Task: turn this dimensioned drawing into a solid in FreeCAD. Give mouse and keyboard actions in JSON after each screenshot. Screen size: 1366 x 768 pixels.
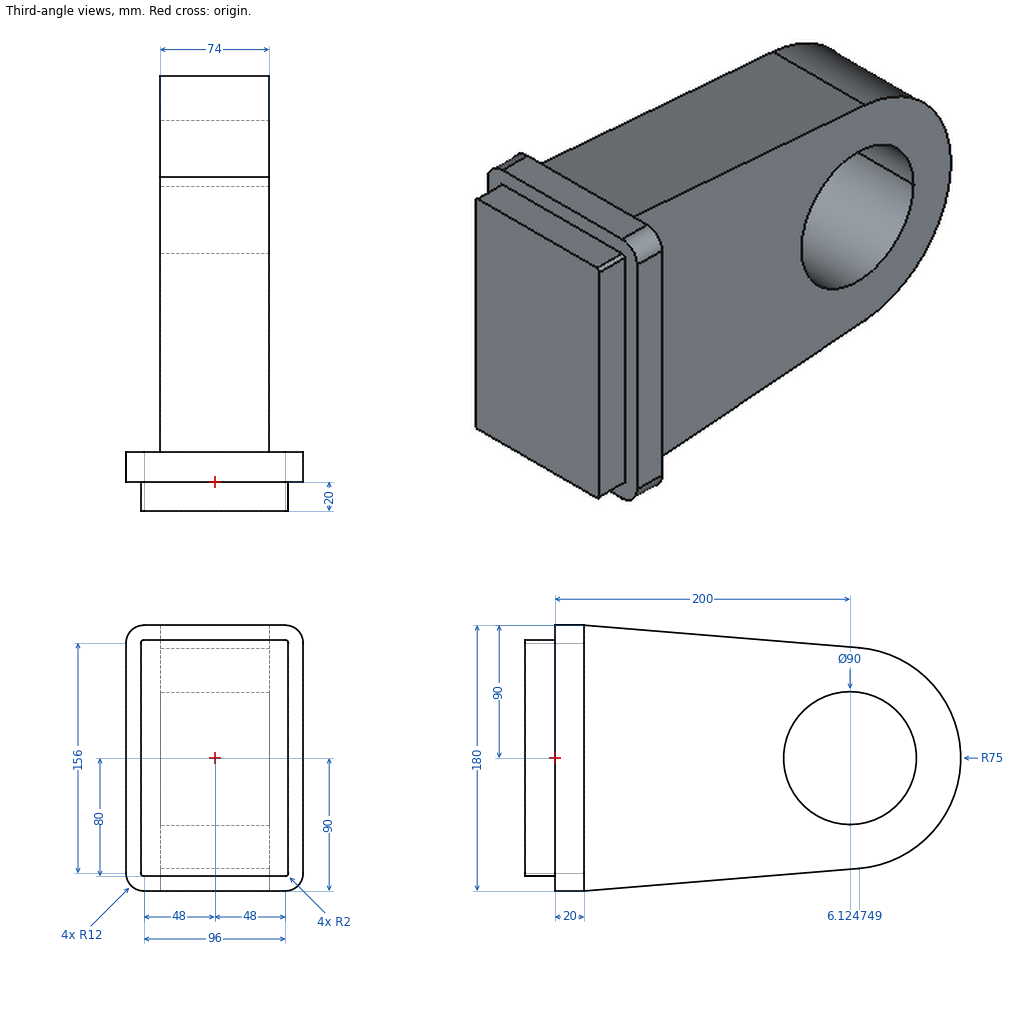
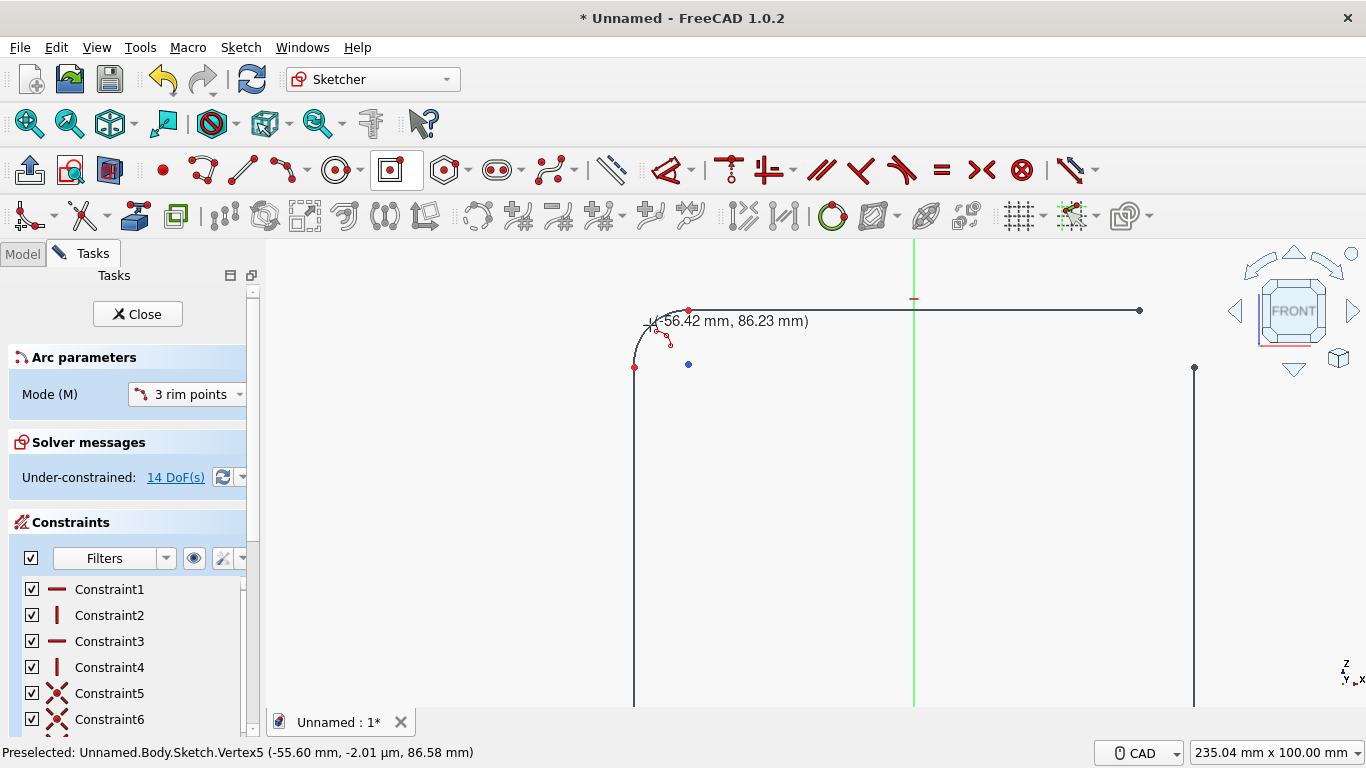
{"action": "left_click", "coordinate": [1140, 310]}
{"action": "left_click", "coordinate": [1194, 367]}
{"action": "left_click", "coordinate": [1178, 325]}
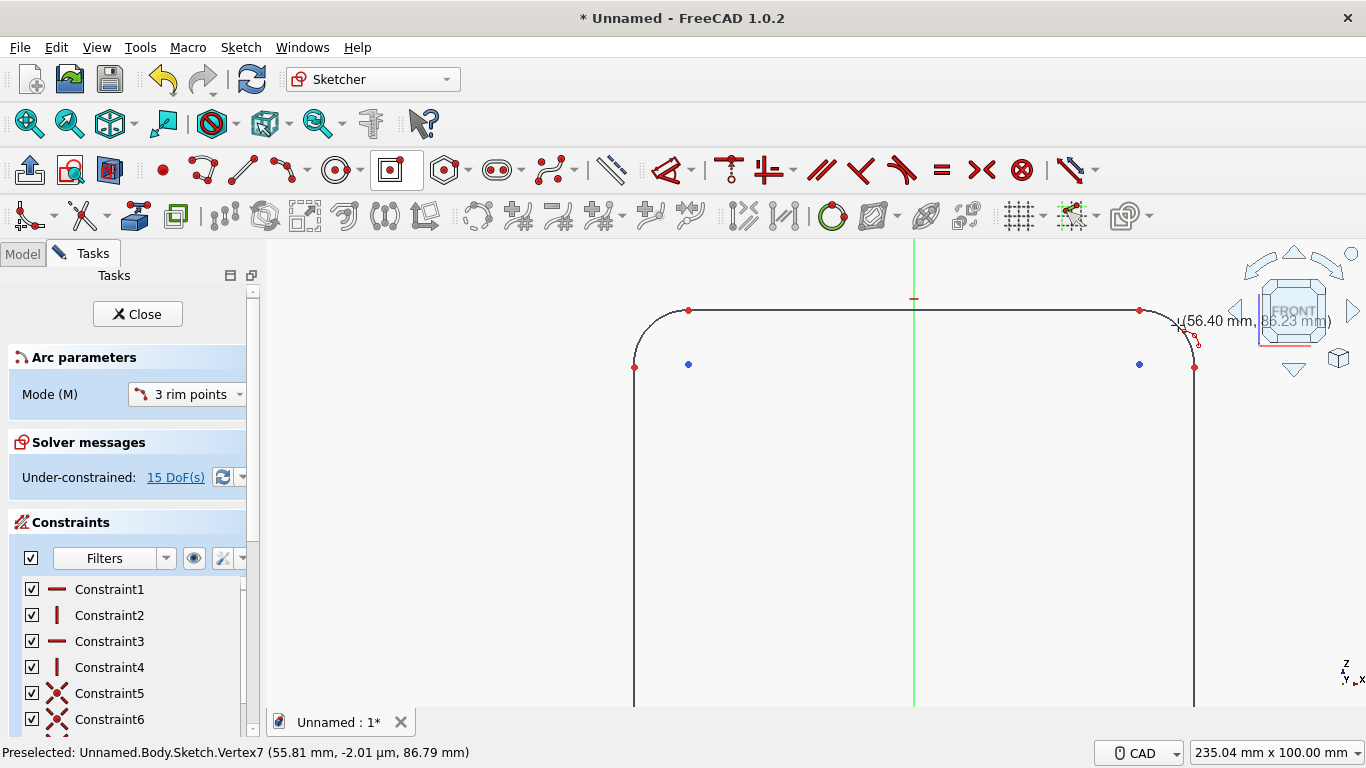
{"action": "scroll", "coordinate": [651, 324], "scroll_direction": "down", "scroll_amount": 5}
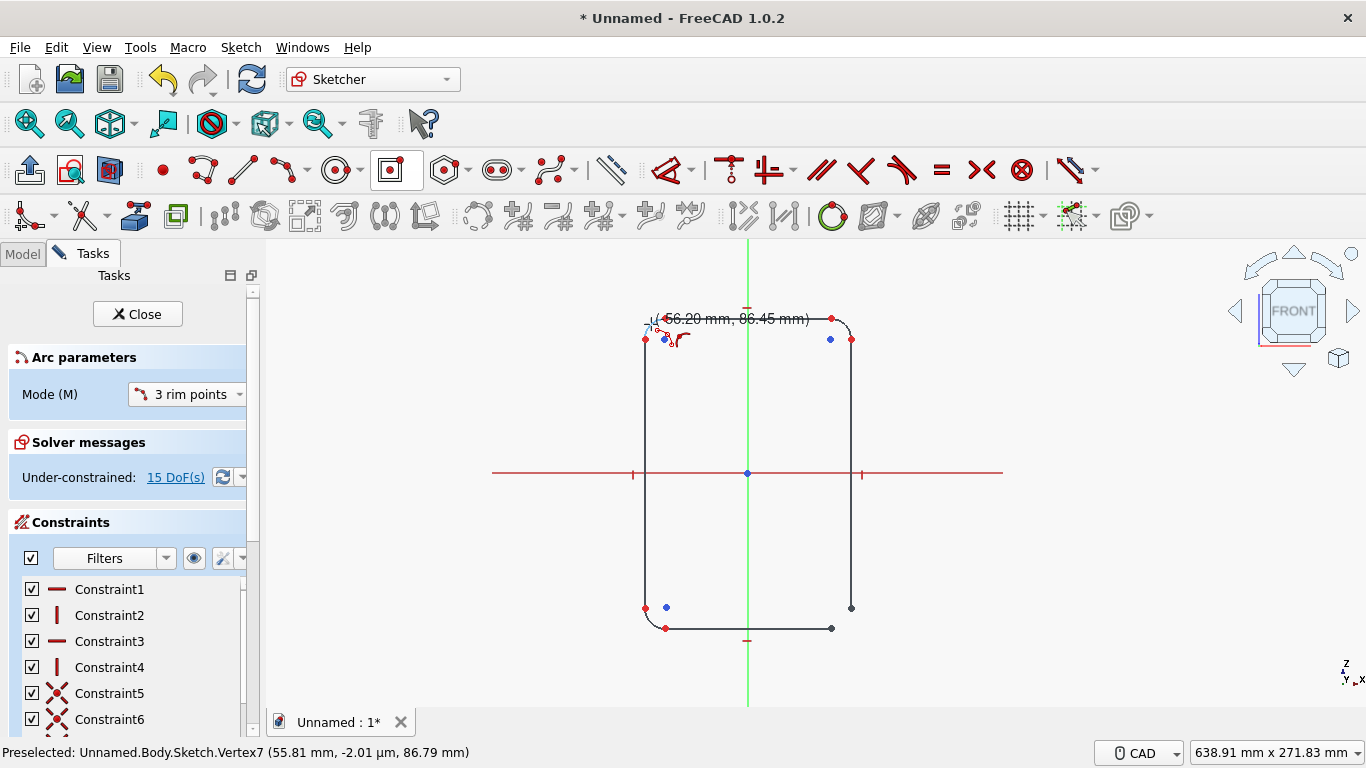
{"action": "left_click", "coordinate": [851, 609]}
{"action": "left_click", "coordinate": [831, 629]}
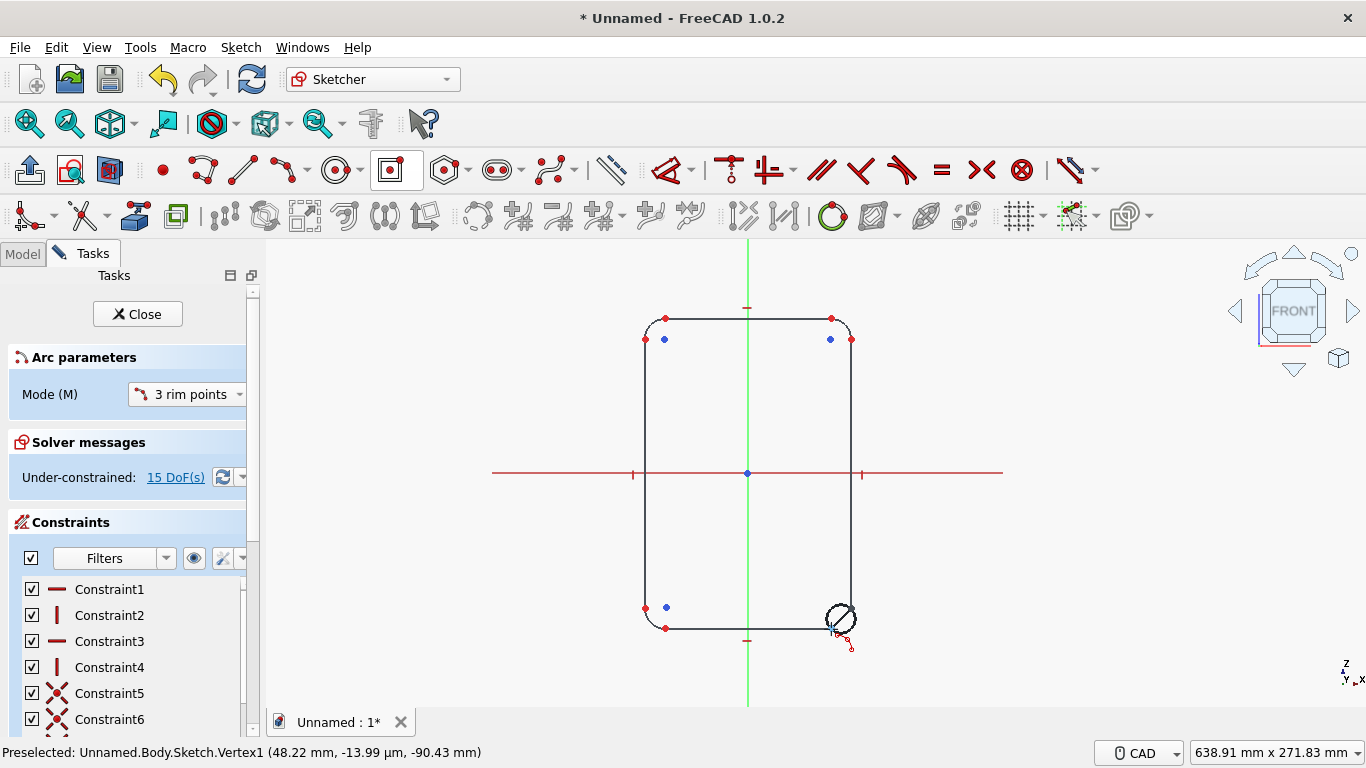
{"action": "scroll", "coordinate": [845, 622], "scroll_direction": "up", "scroll_amount": 5}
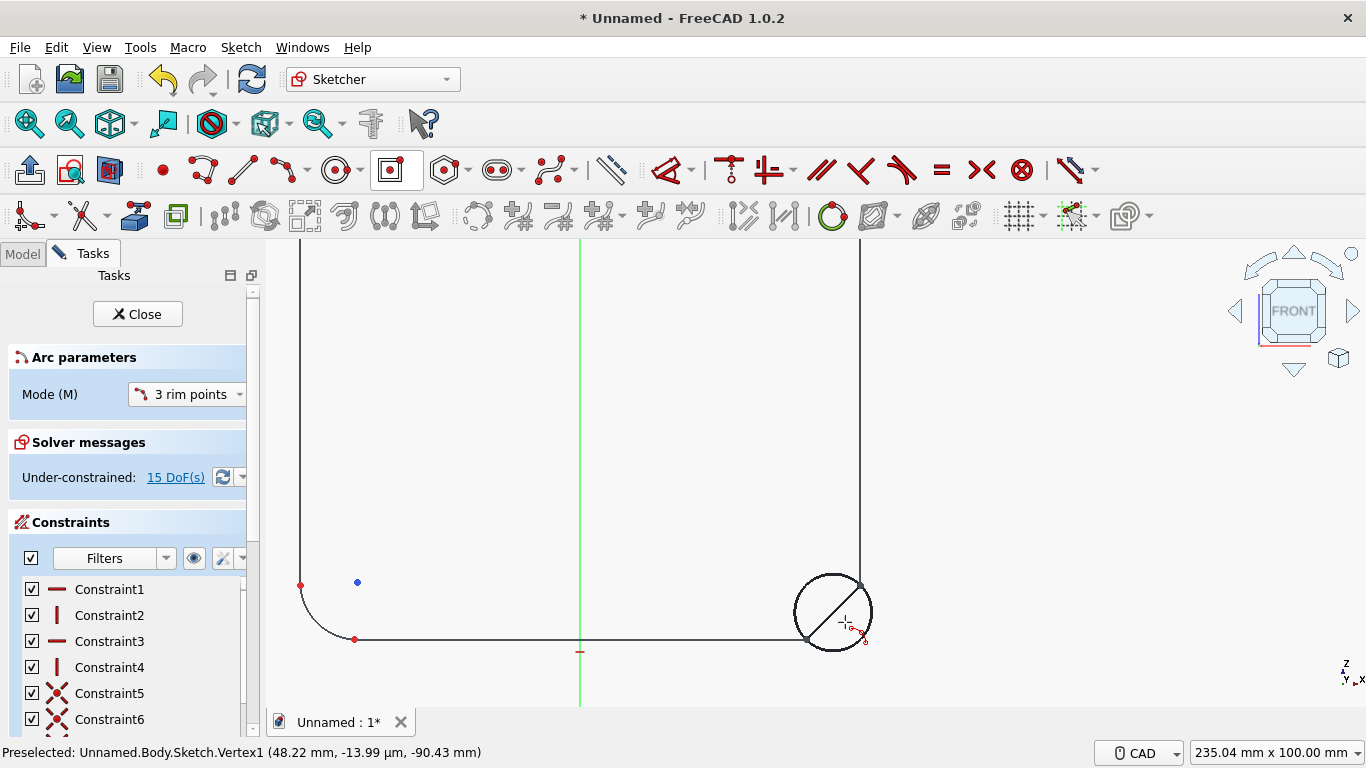
{"action": "left_click", "coordinate": [845, 621]}
{"action": "key", "text": "Escape"}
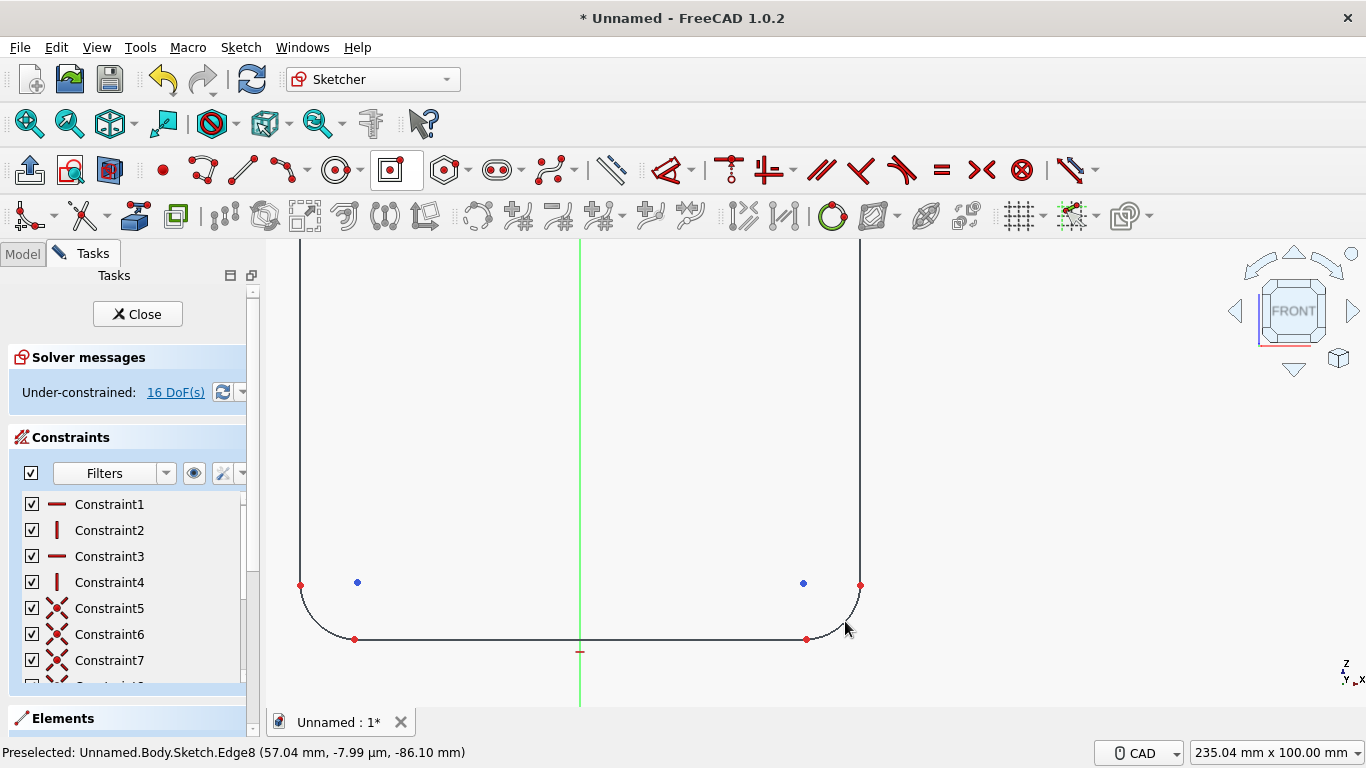
{"action": "left_click", "coordinate": [671, 640]}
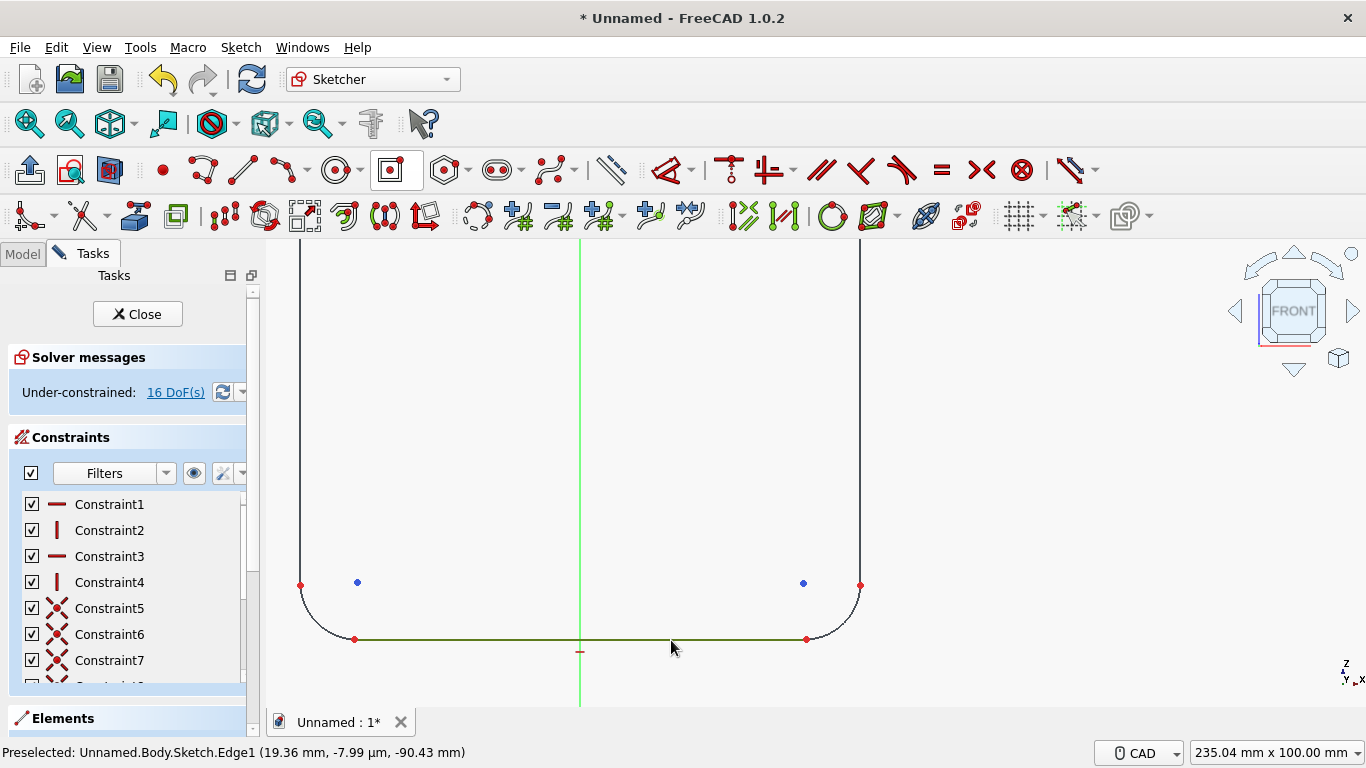
{"action": "left_click", "coordinate": [307, 609]}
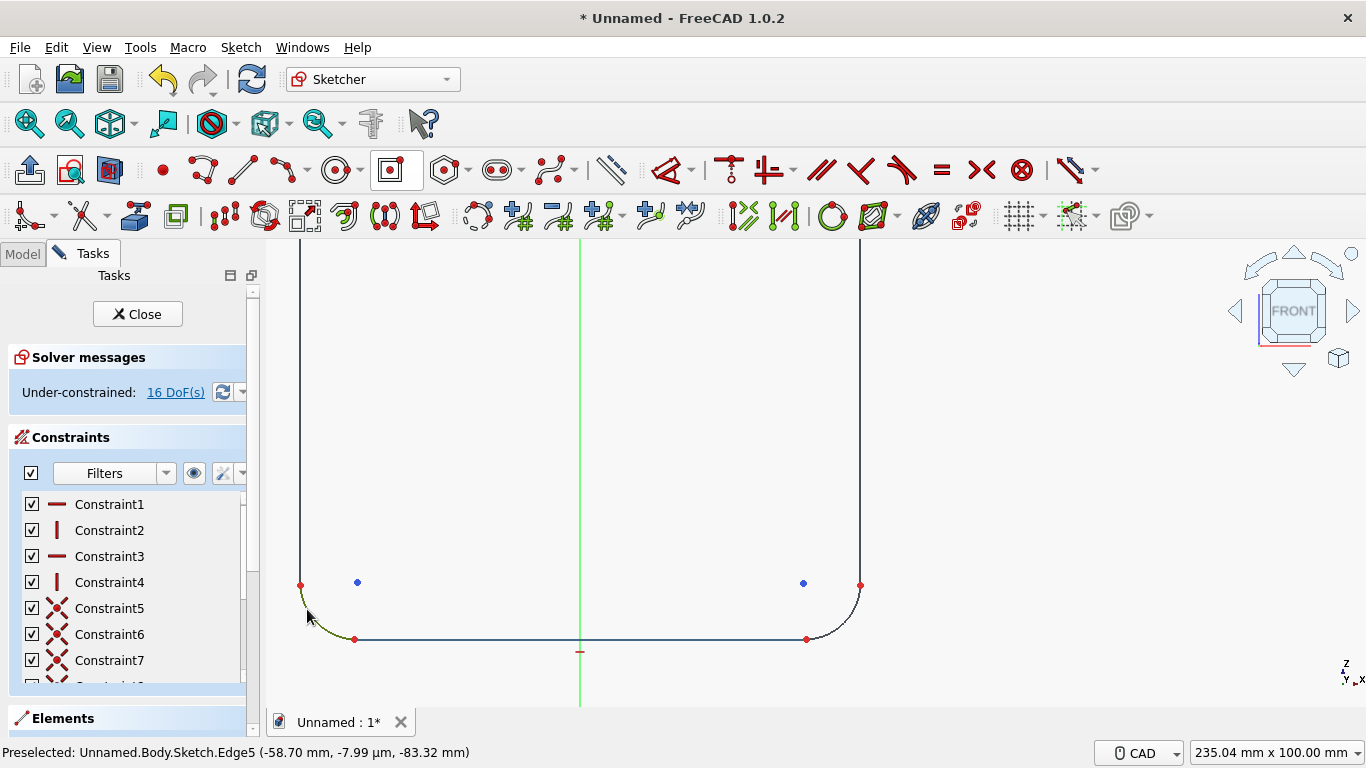
{"action": "key", "text": "t"}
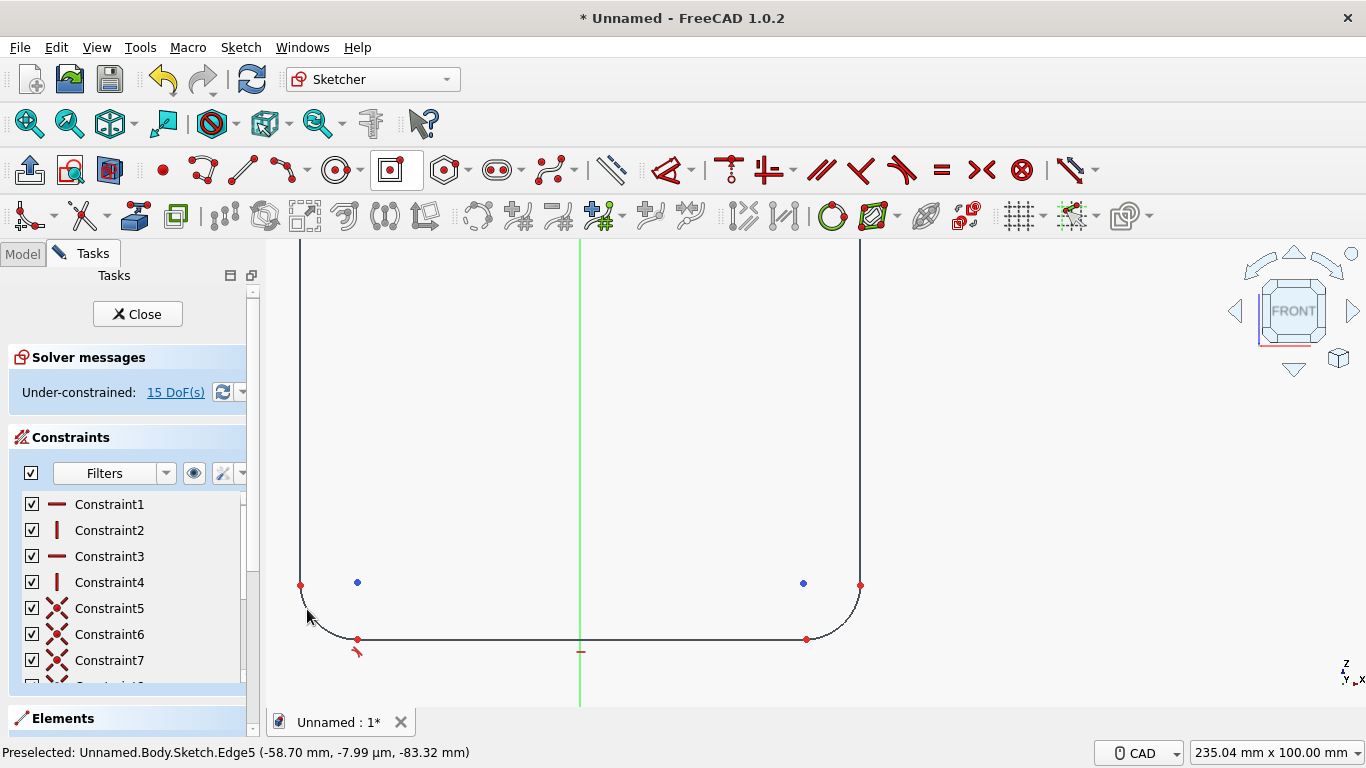
{"action": "left_click", "coordinate": [672, 640]}